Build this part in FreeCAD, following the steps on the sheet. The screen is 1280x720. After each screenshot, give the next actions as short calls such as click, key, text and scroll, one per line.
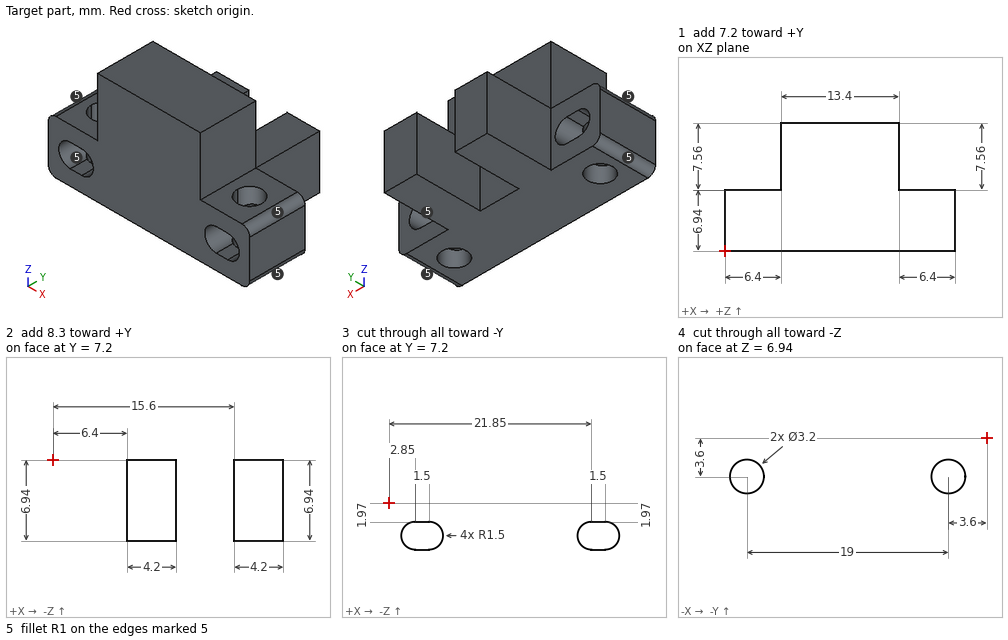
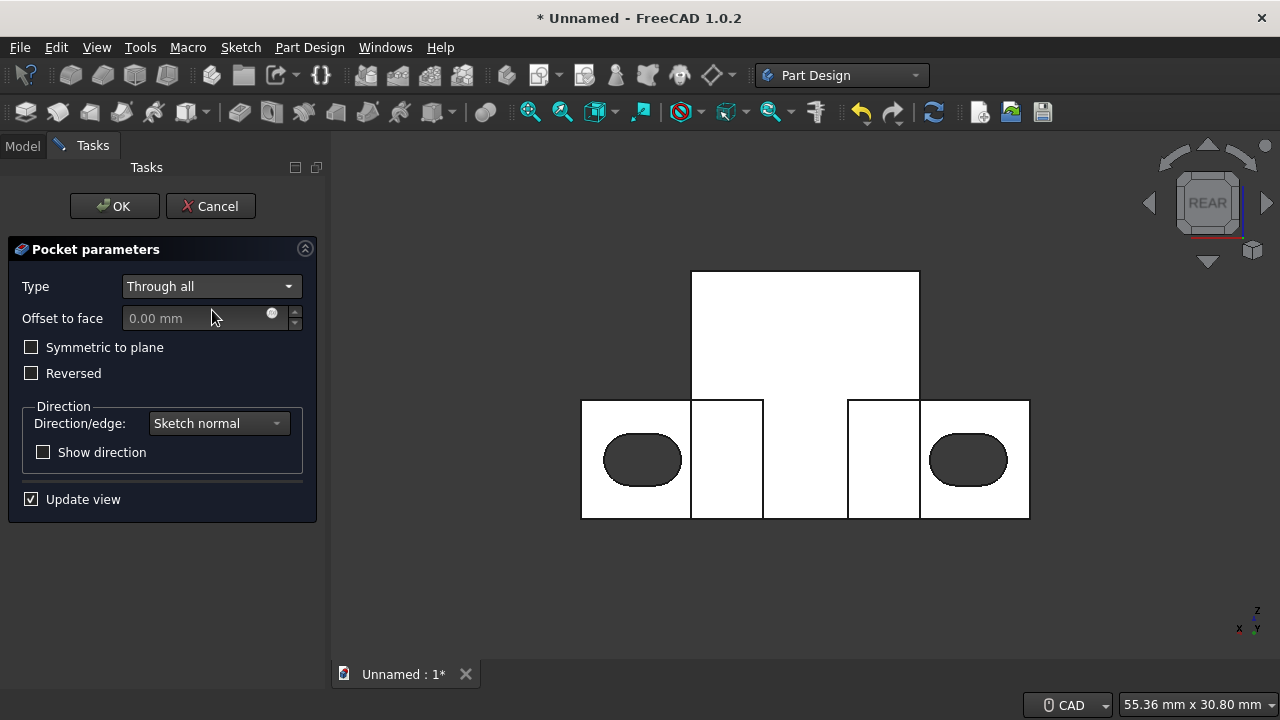
click(115, 206)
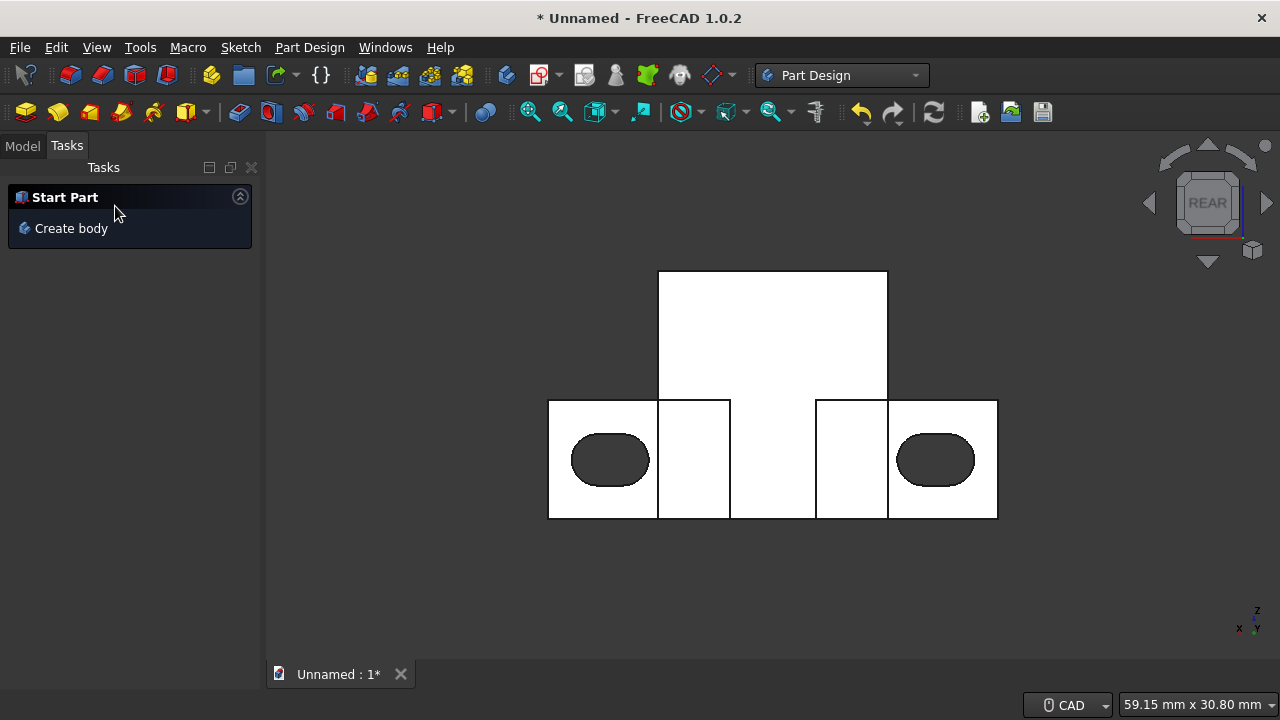
key(0)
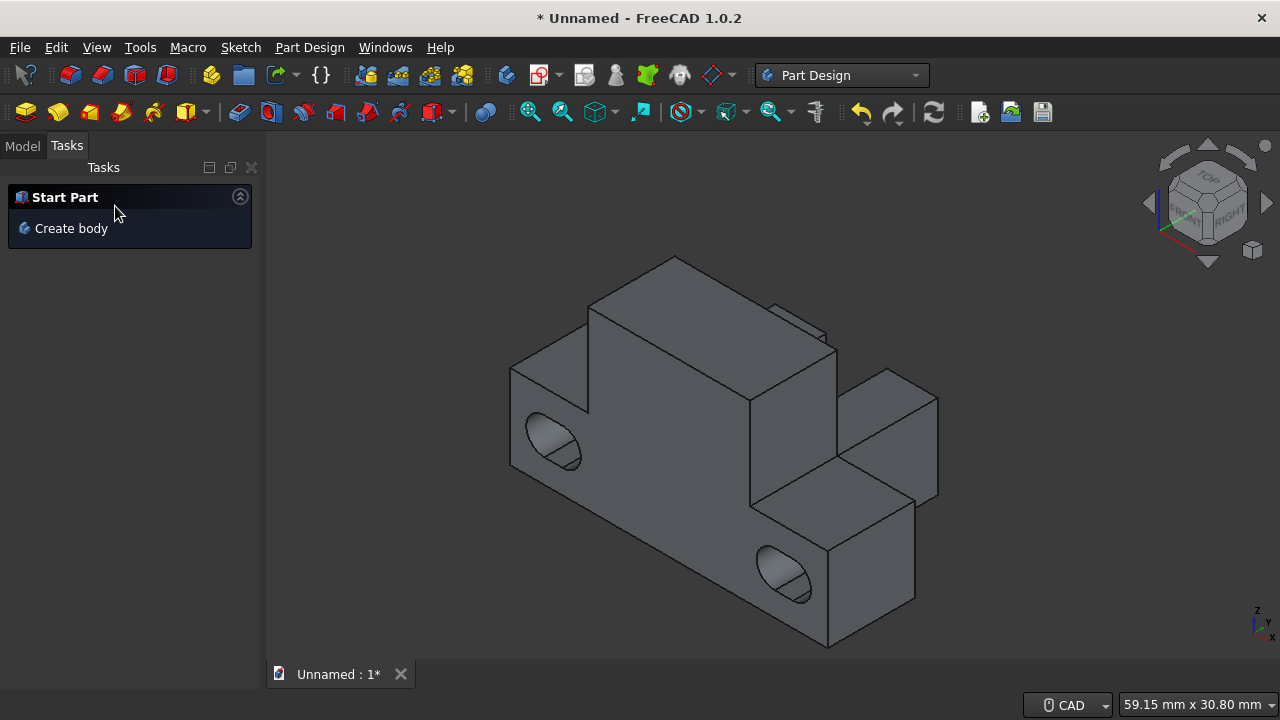
click(832, 503)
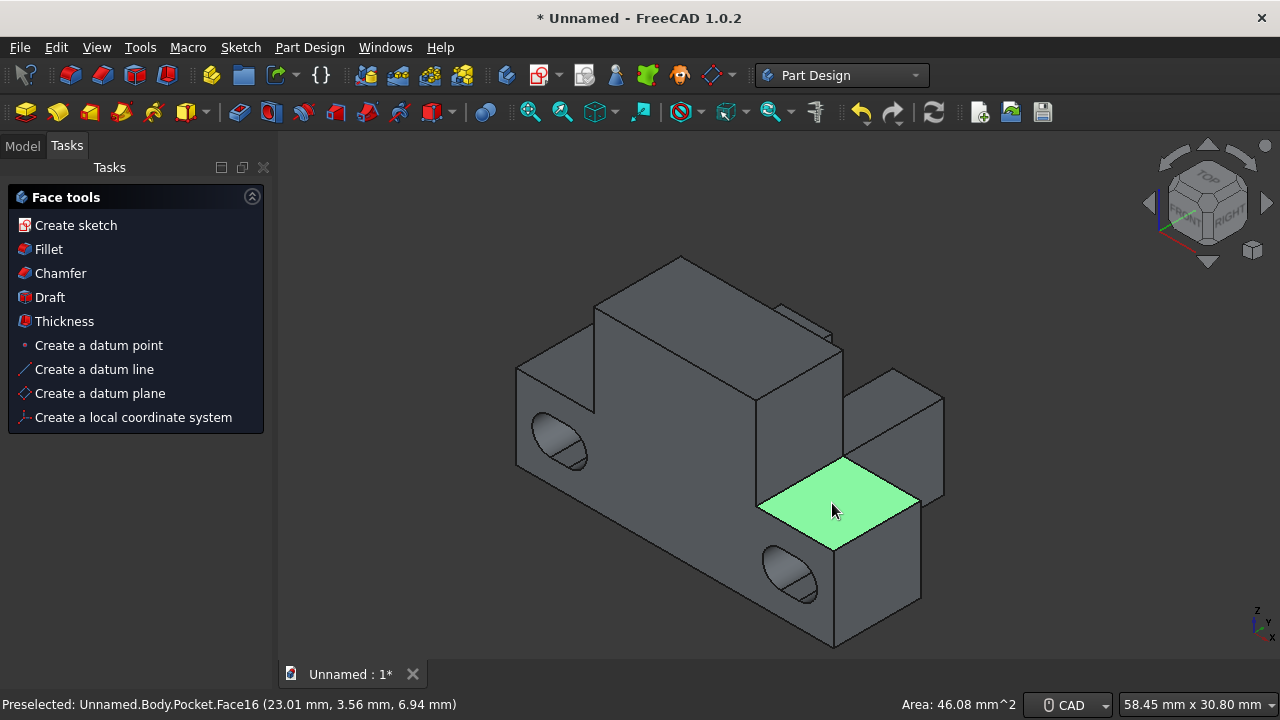
click(540, 76)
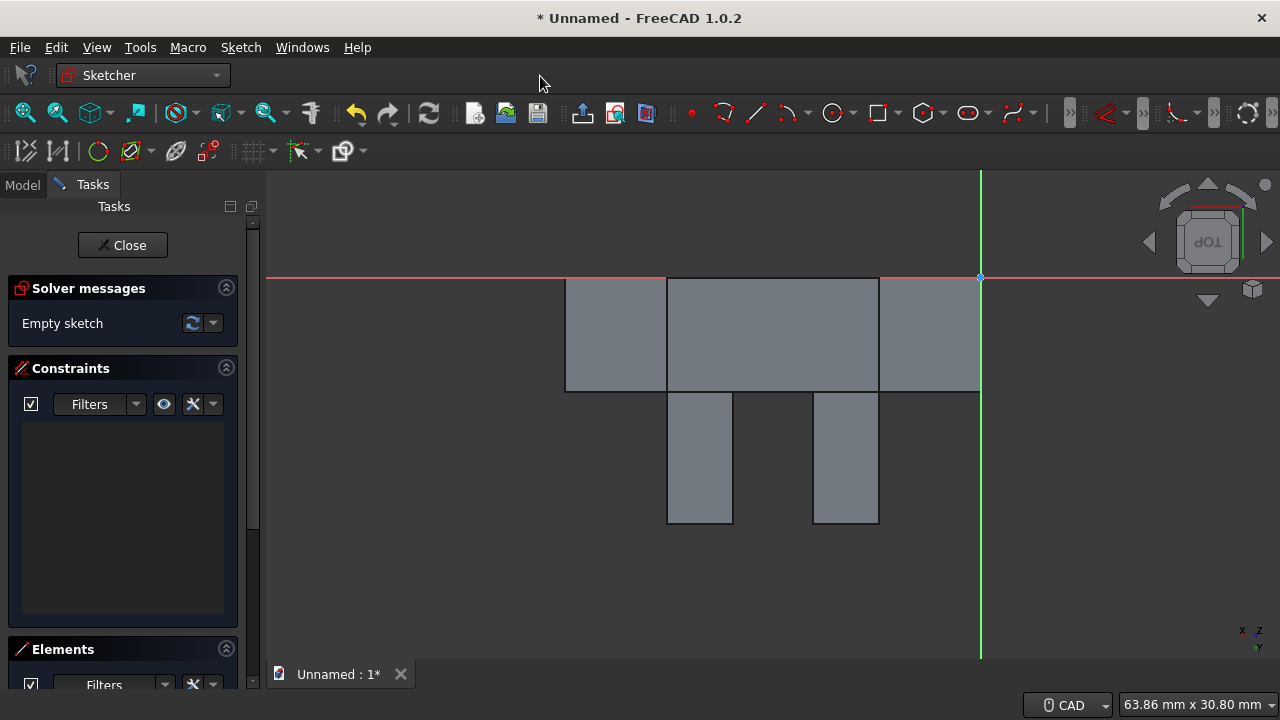
scroll(960, 198, up, 2)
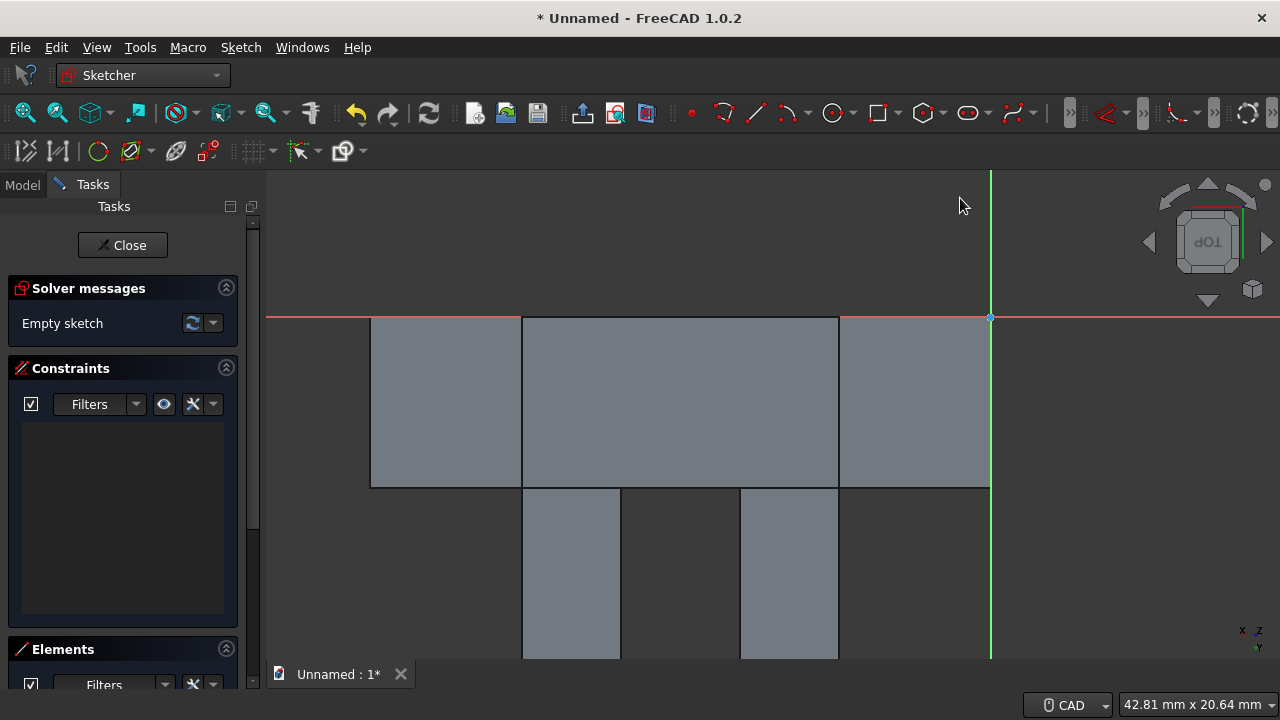
click(834, 114)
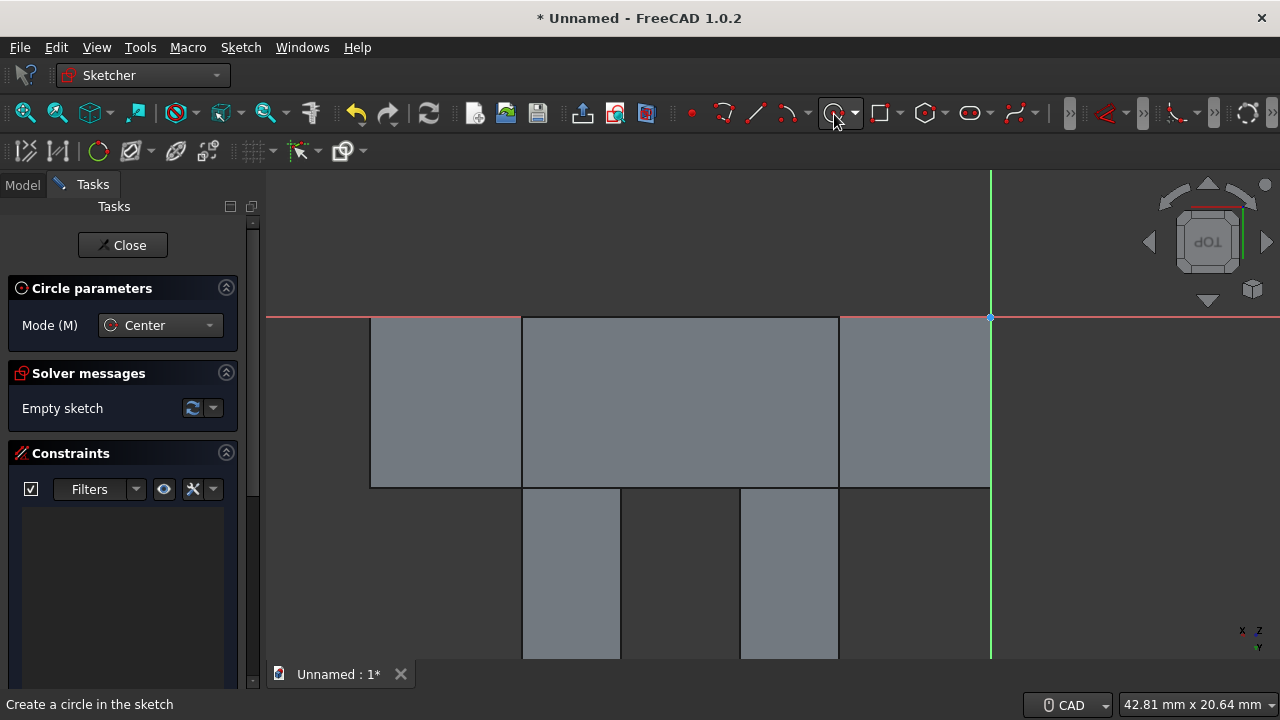
click(456, 403)
click(482, 376)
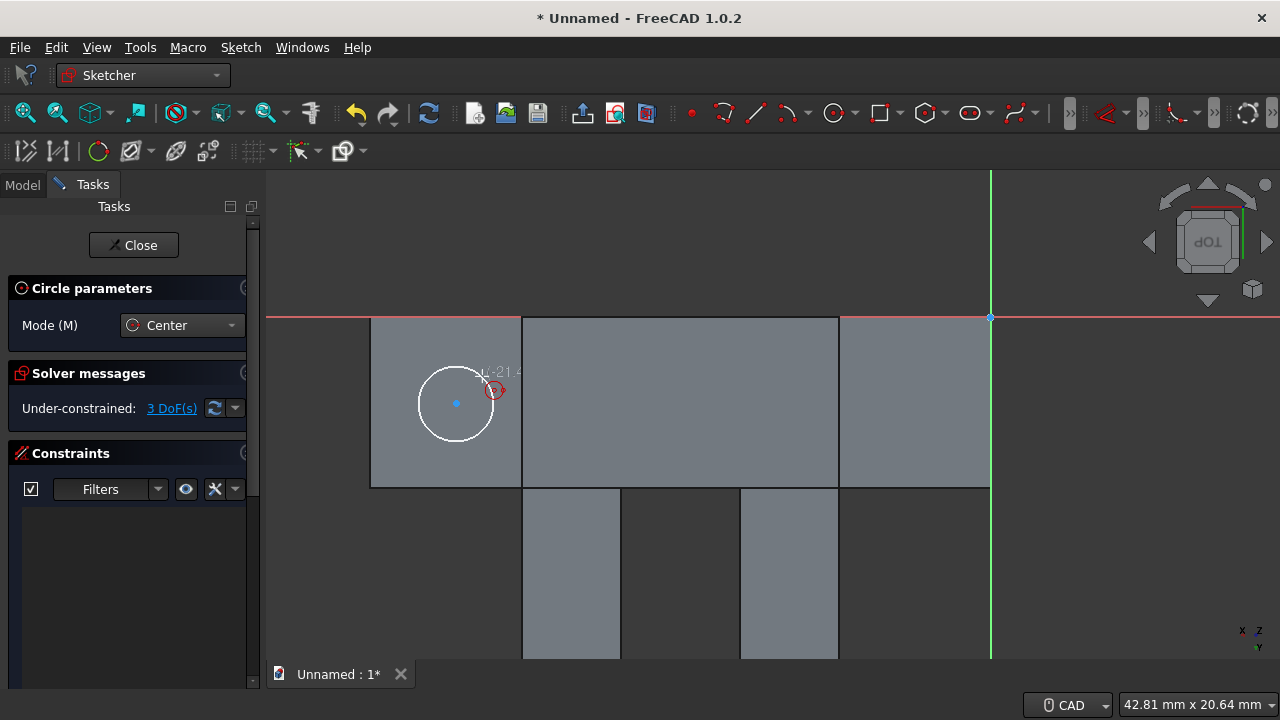
click(906, 403)
click(933, 376)
key(Escape)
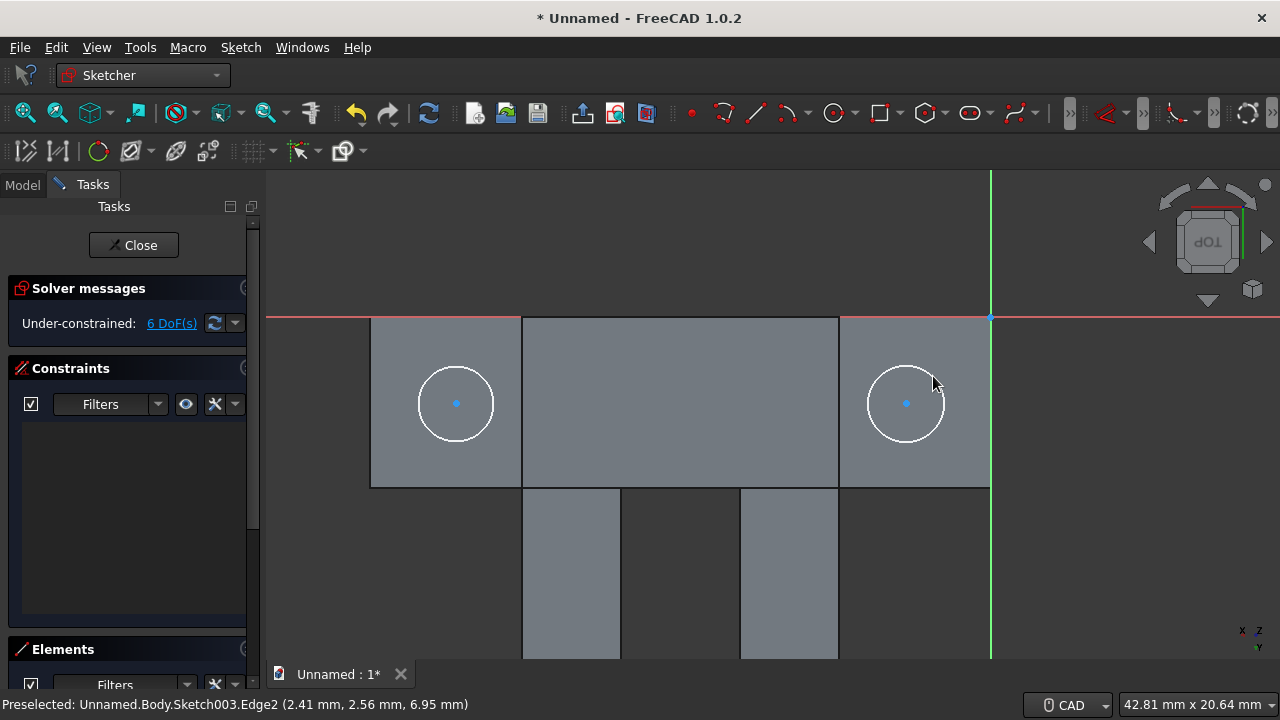
click(482, 377)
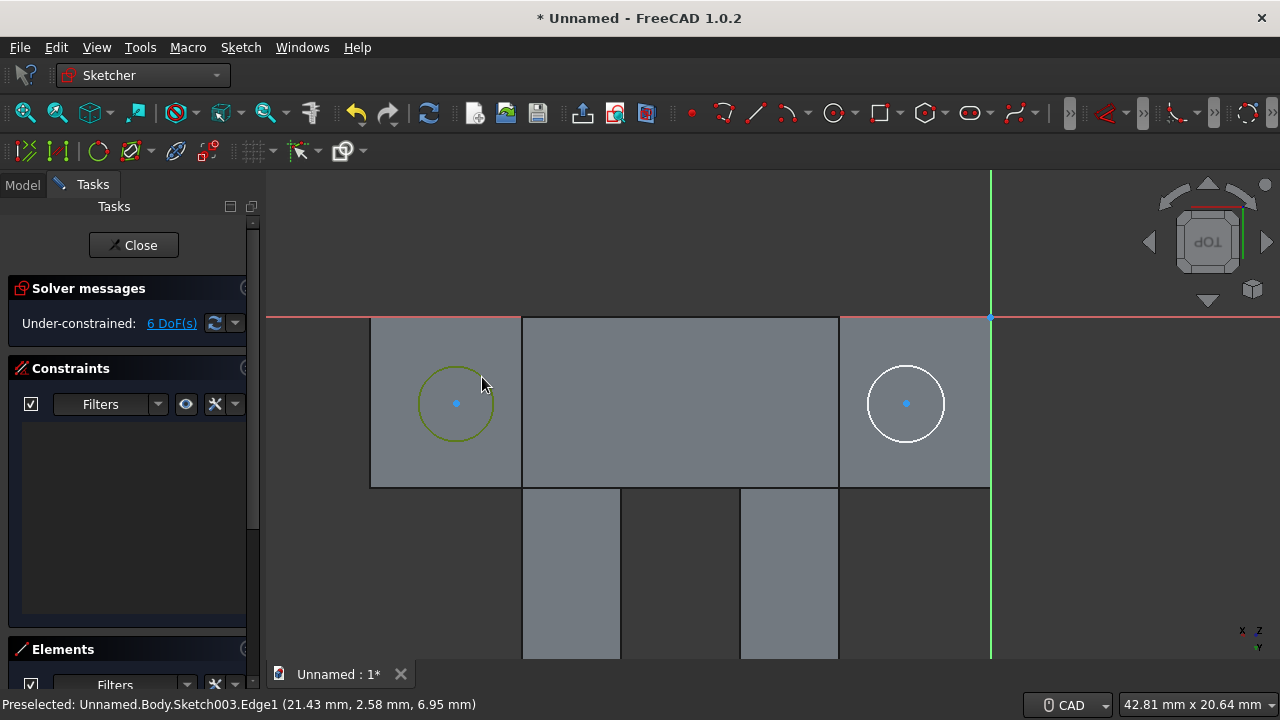
click(933, 377)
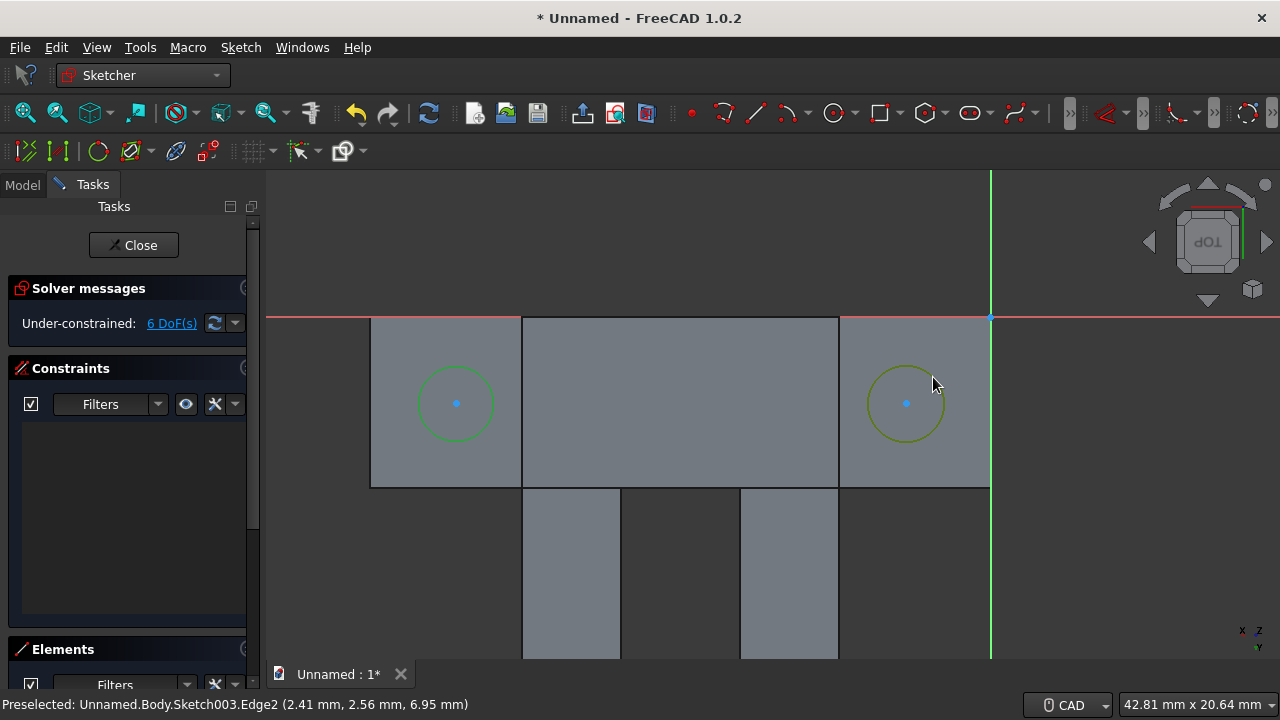
key(e)